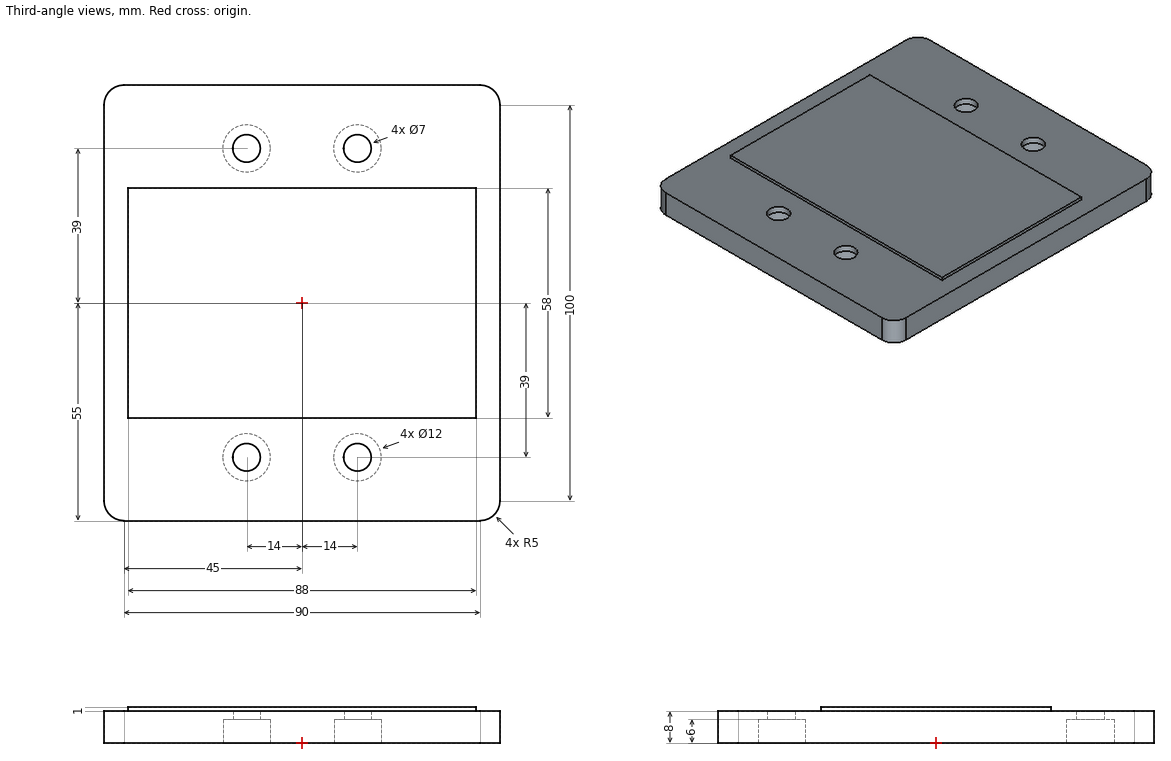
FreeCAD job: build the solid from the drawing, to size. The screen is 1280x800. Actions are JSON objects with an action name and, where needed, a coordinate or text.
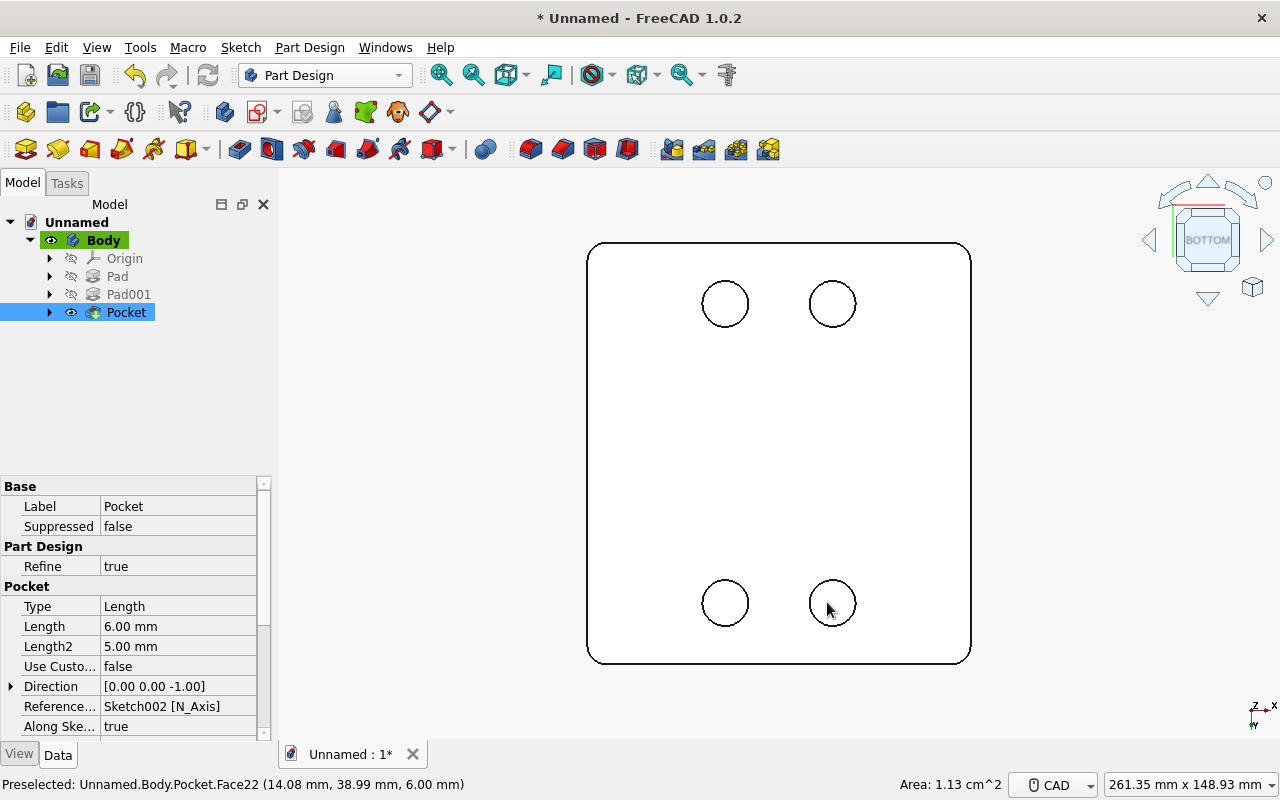
{"action": "left_click", "coordinate": [258, 112]}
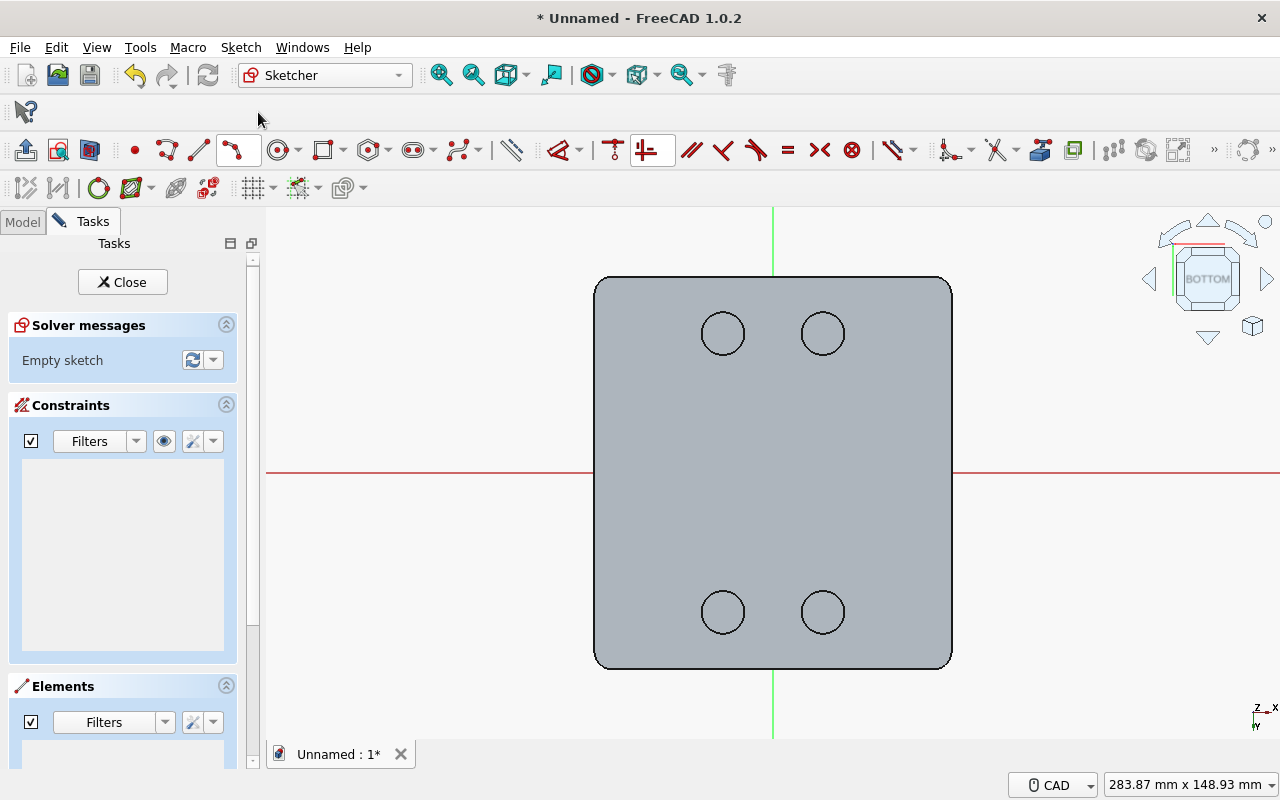
{"action": "key", "text": "q s"}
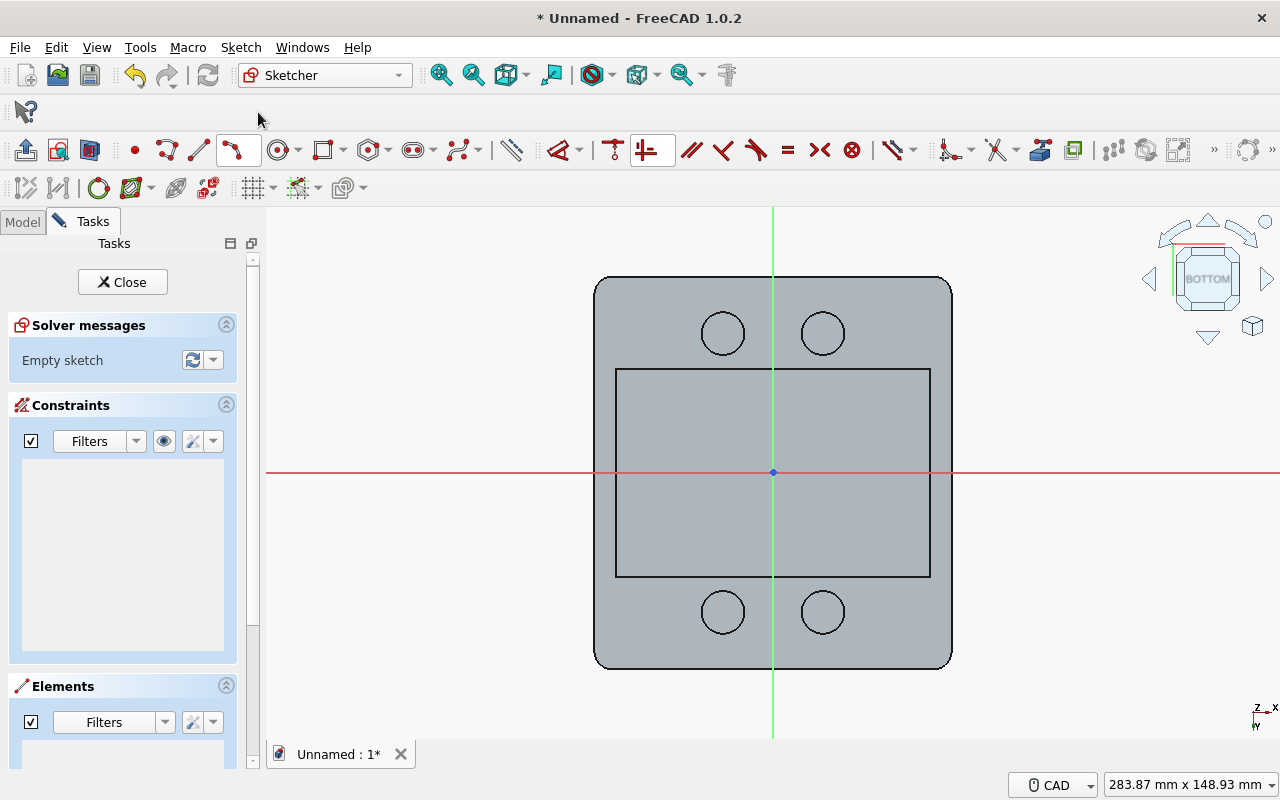
{"action": "key", "text": "g c"}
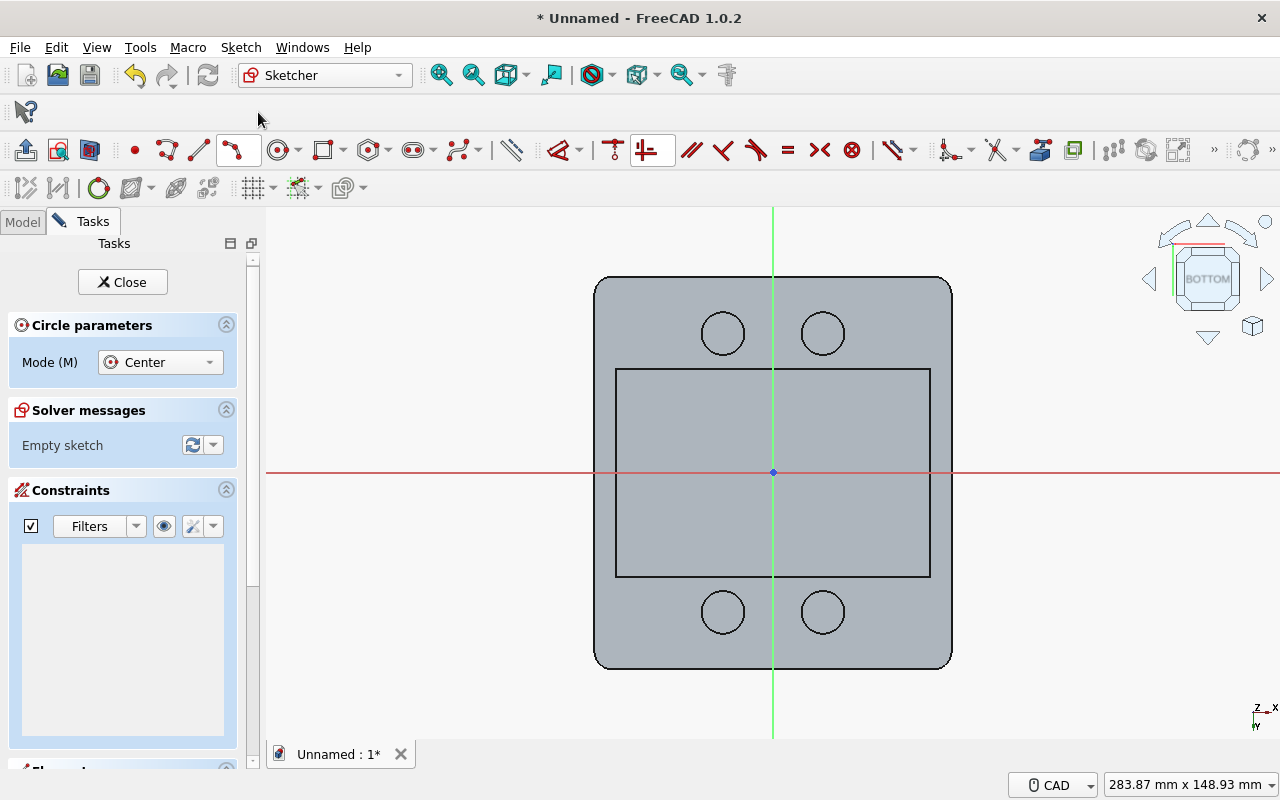
{"action": "scroll", "coordinate": [823, 612], "scroll_direction": "up", "scroll_amount": 3}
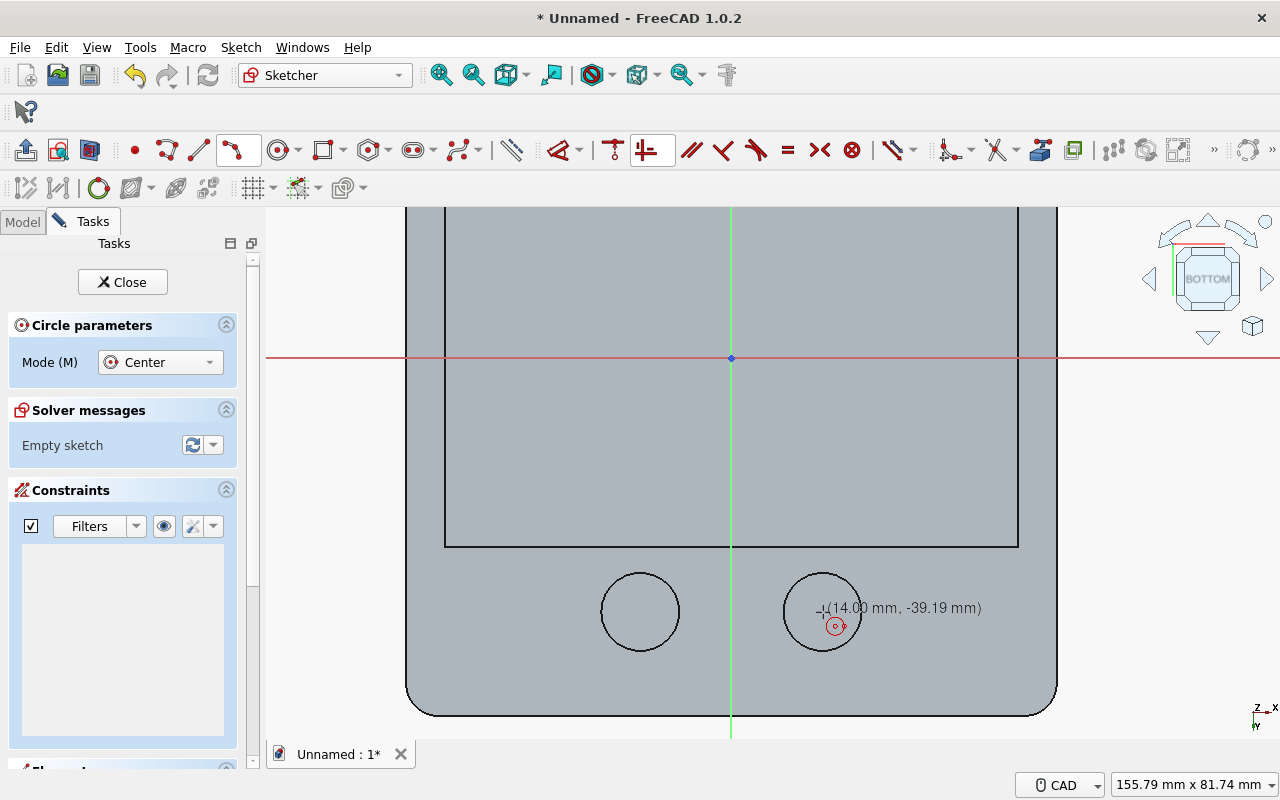
{"action": "left_click", "coordinate": [823, 612]}
{"action": "mouse_move", "coordinate": [839, 596]}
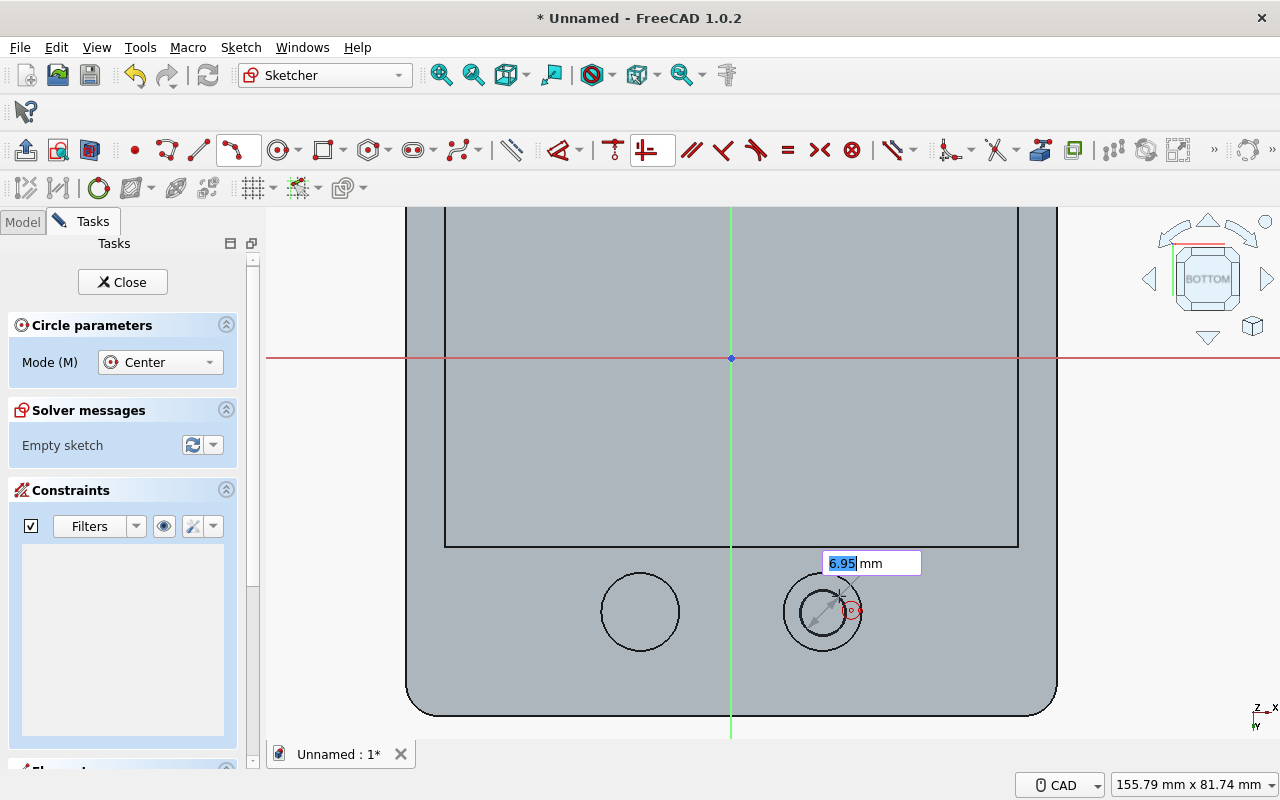
{"action": "type", "text": "7"}
{"action": "key", "text": "Return"}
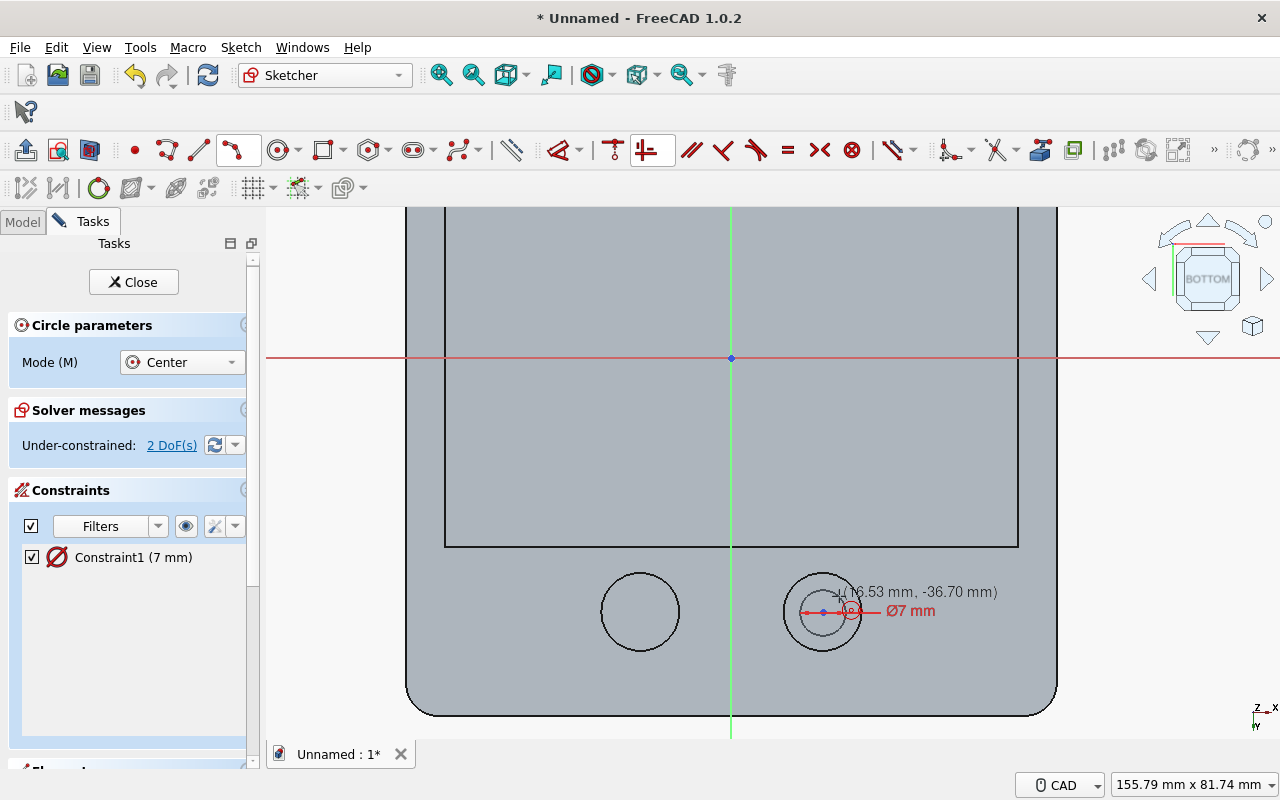
{"action": "left_click", "coordinate": [640, 612]}
{"action": "mouse_move", "coordinate": [656, 596]}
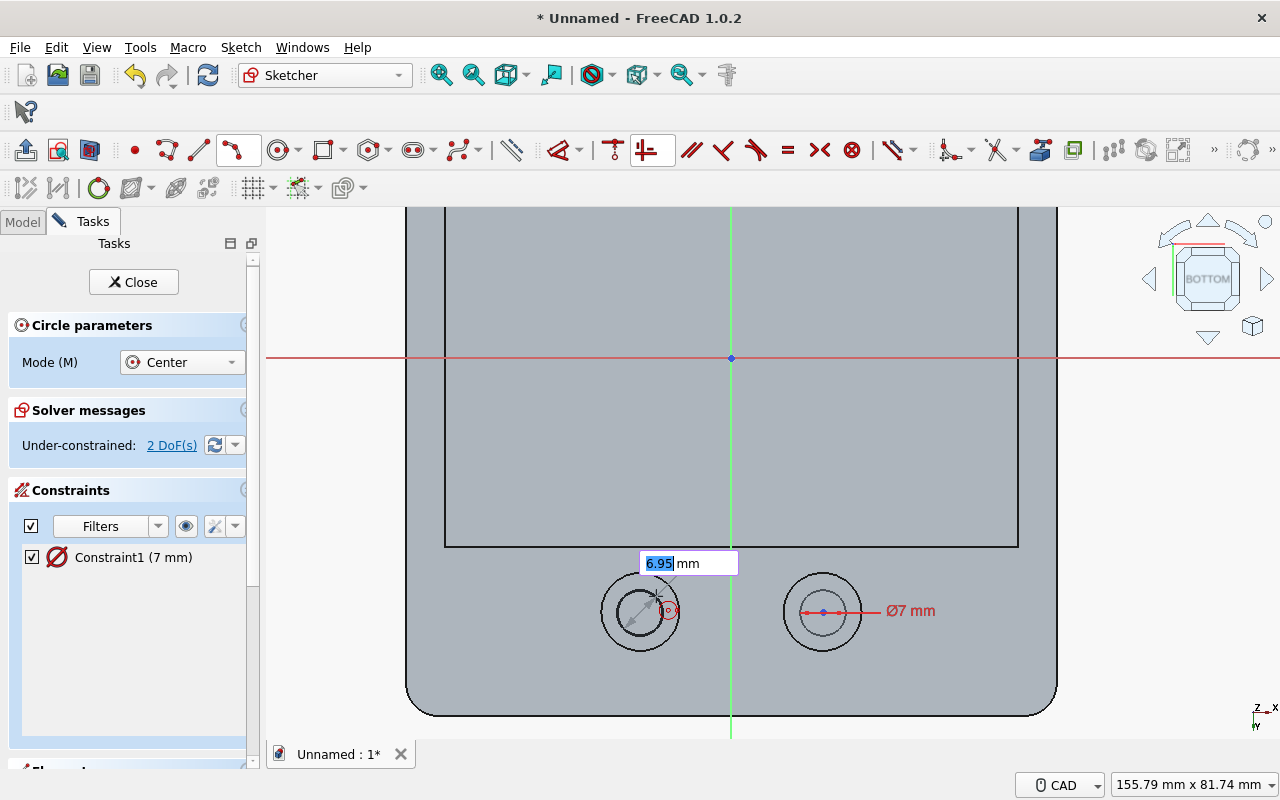
{"action": "type", "text": "7"}
{"action": "key", "text": "Return"}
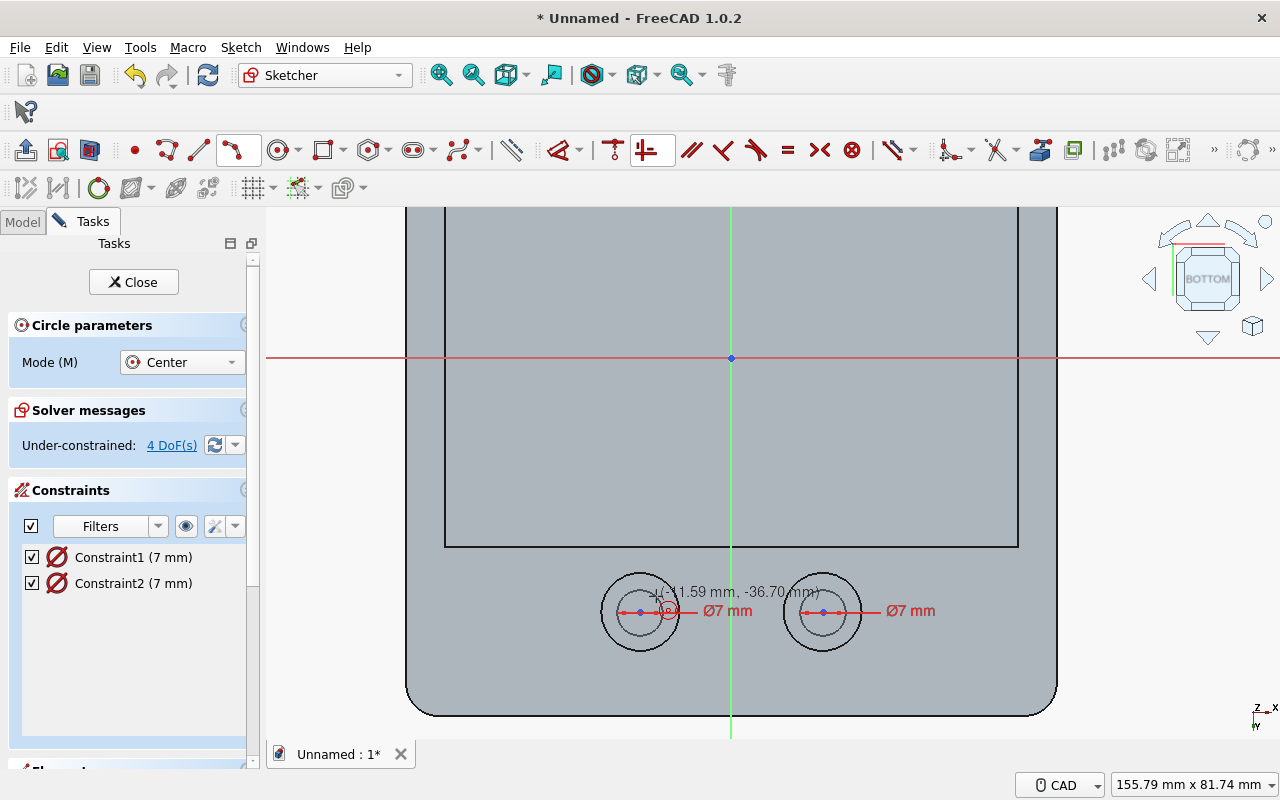
{"action": "scroll", "coordinate": [650, 707], "scroll_direction": "down", "scroll_amount": 2}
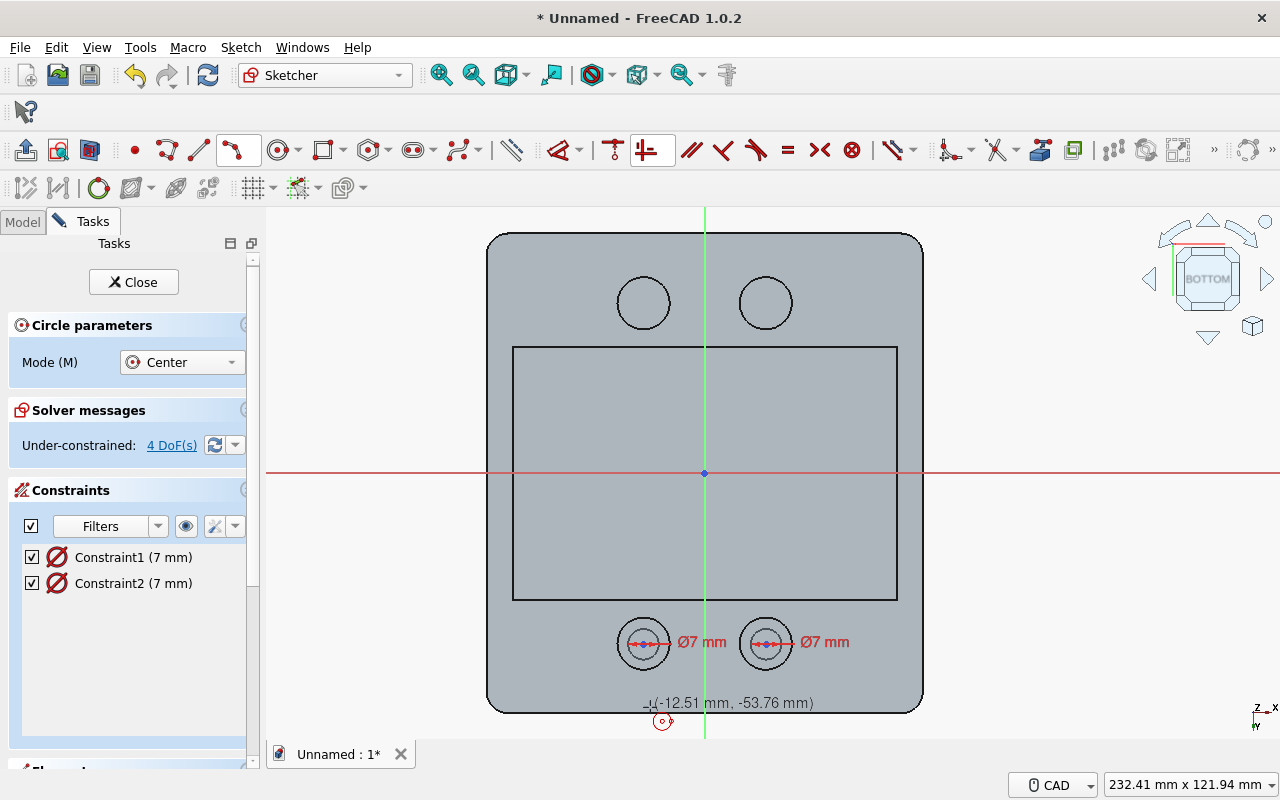
{"action": "scroll", "coordinate": [644, 303], "scroll_direction": "up", "scroll_amount": 2}